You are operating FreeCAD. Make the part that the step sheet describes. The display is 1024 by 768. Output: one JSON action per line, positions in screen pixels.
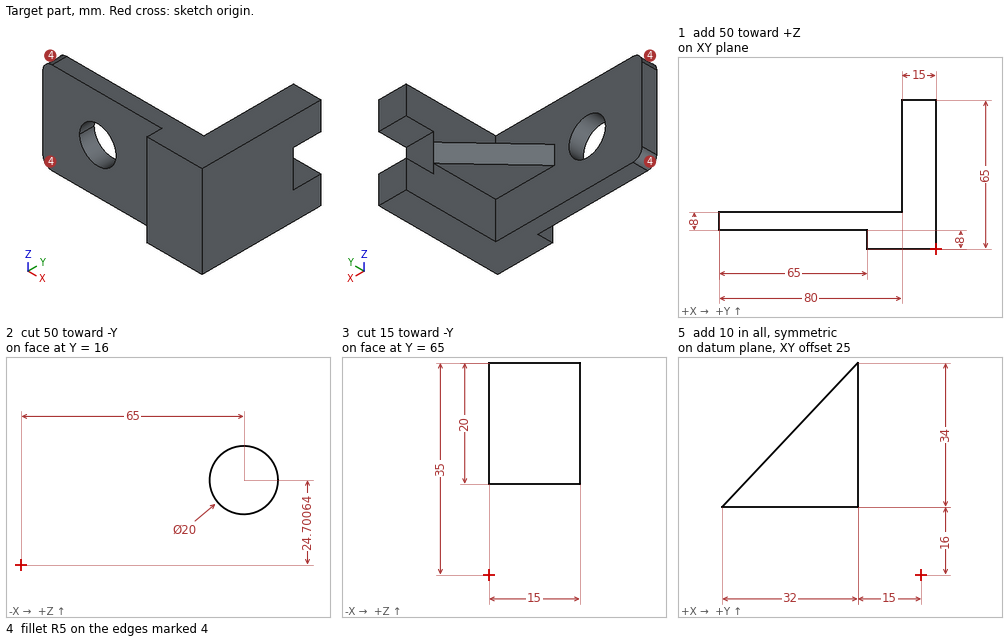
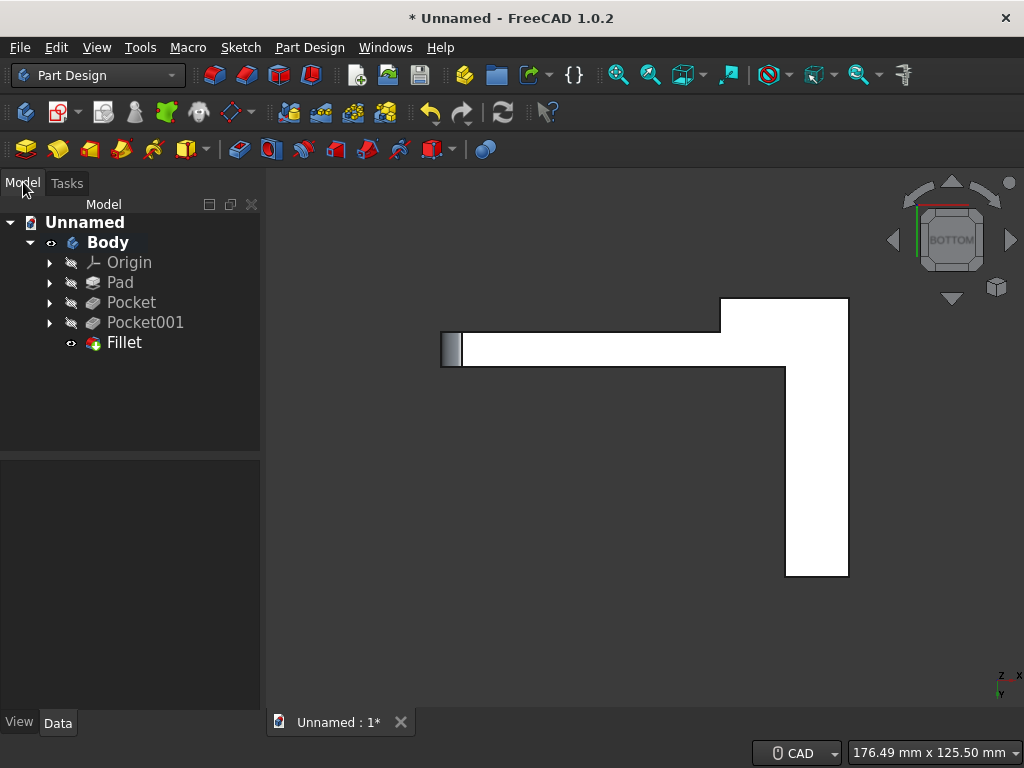
{"action": "left_click", "coordinate": [50, 263]}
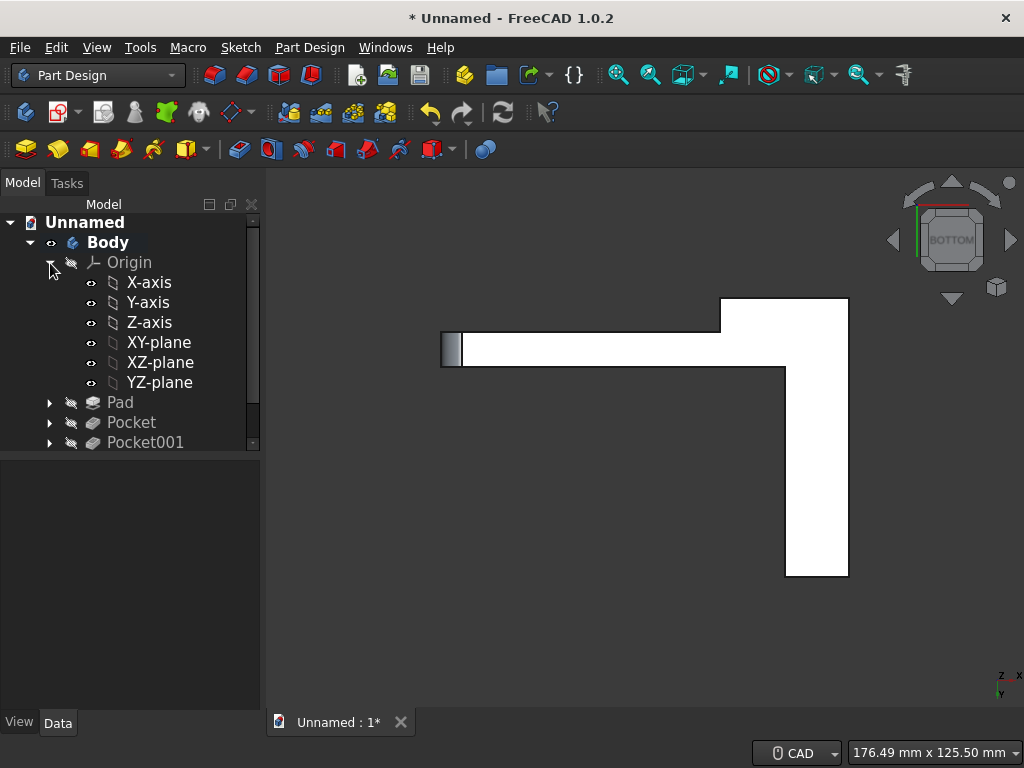
{"action": "left_click", "coordinate": [136, 343]}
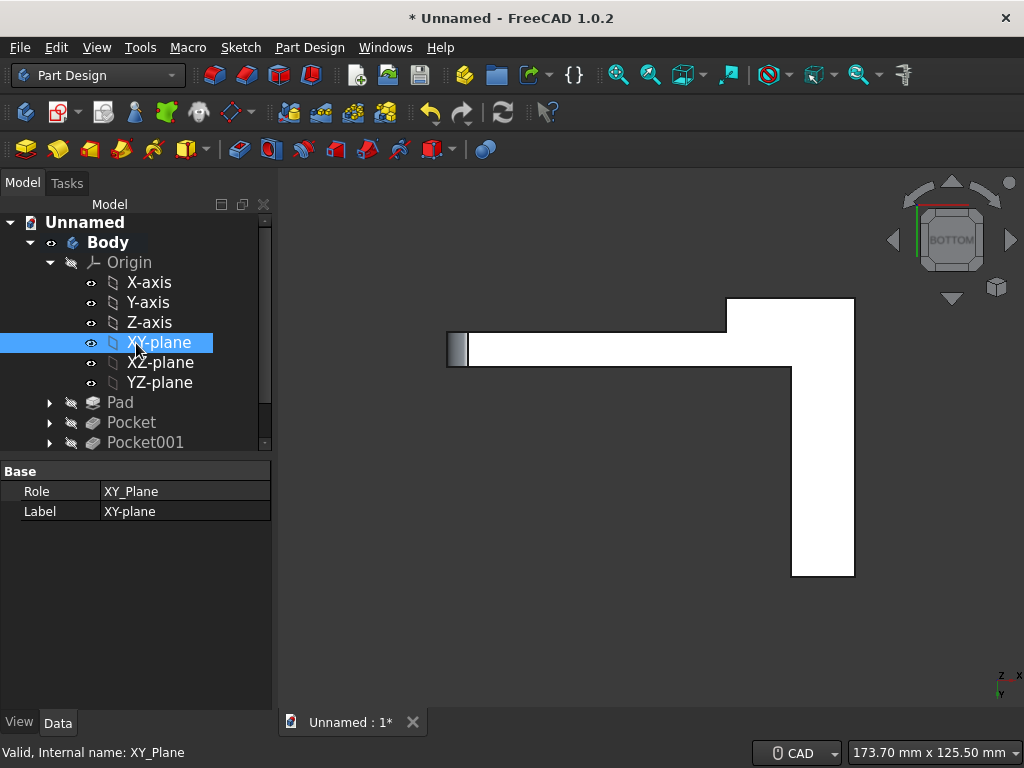
{"action": "left_click", "coordinate": [232, 112]}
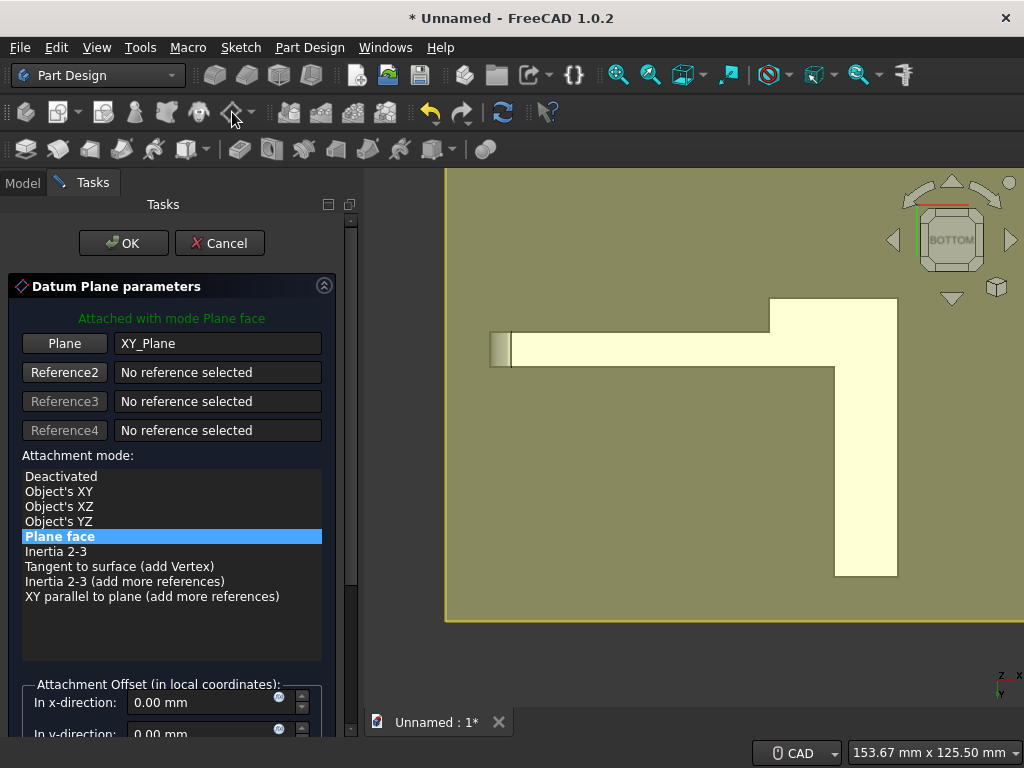
{"action": "scroll", "coordinate": [351, 475], "scroll_direction": "down", "scroll_amount": 2}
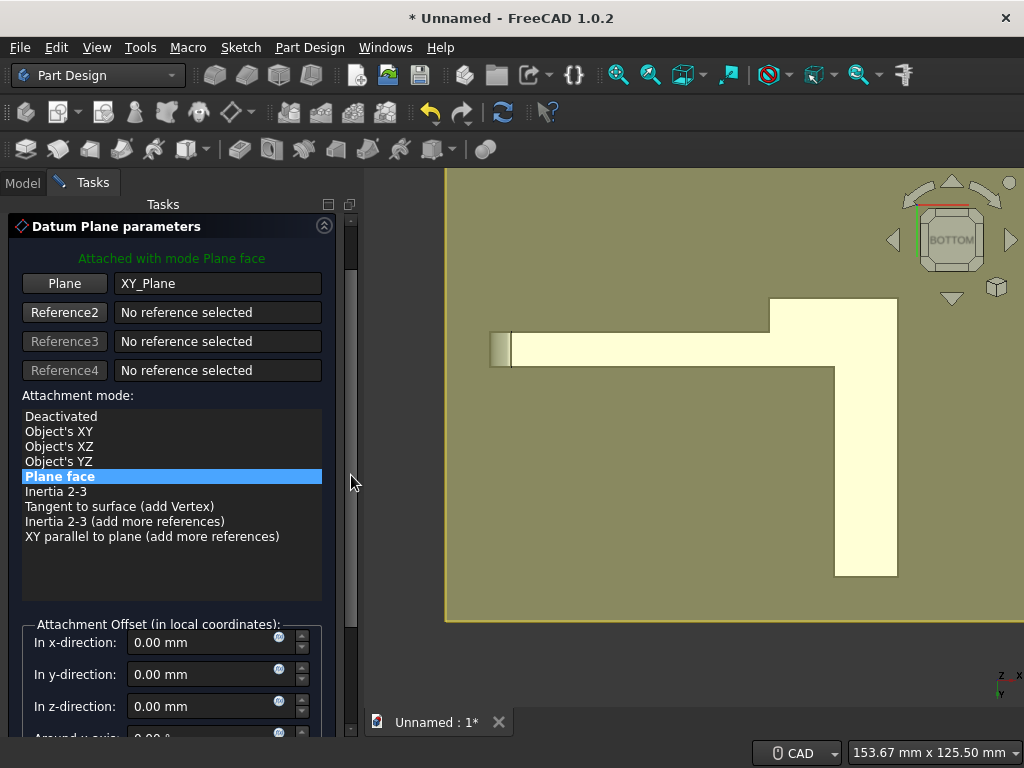
{"action": "triple_click", "coordinate": [210, 646]}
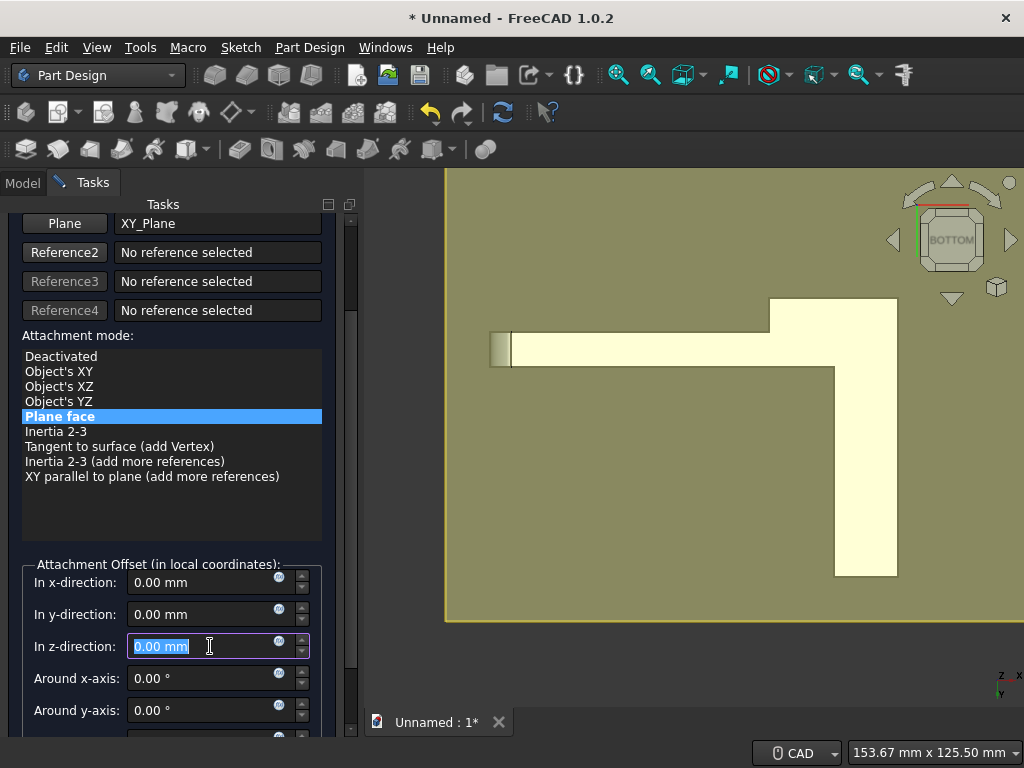
{"action": "type", "text": "25"}
{"action": "key", "text": "Tab"}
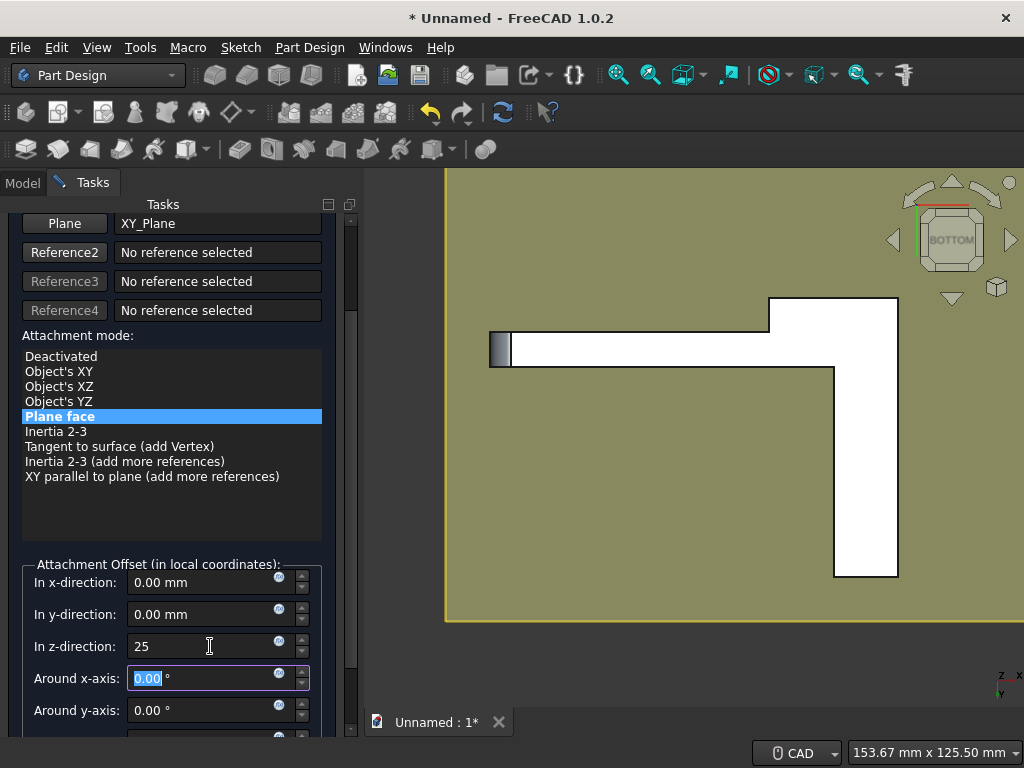
{"action": "scroll", "coordinate": [351, 475], "scroll_direction": "up", "scroll_amount": 3}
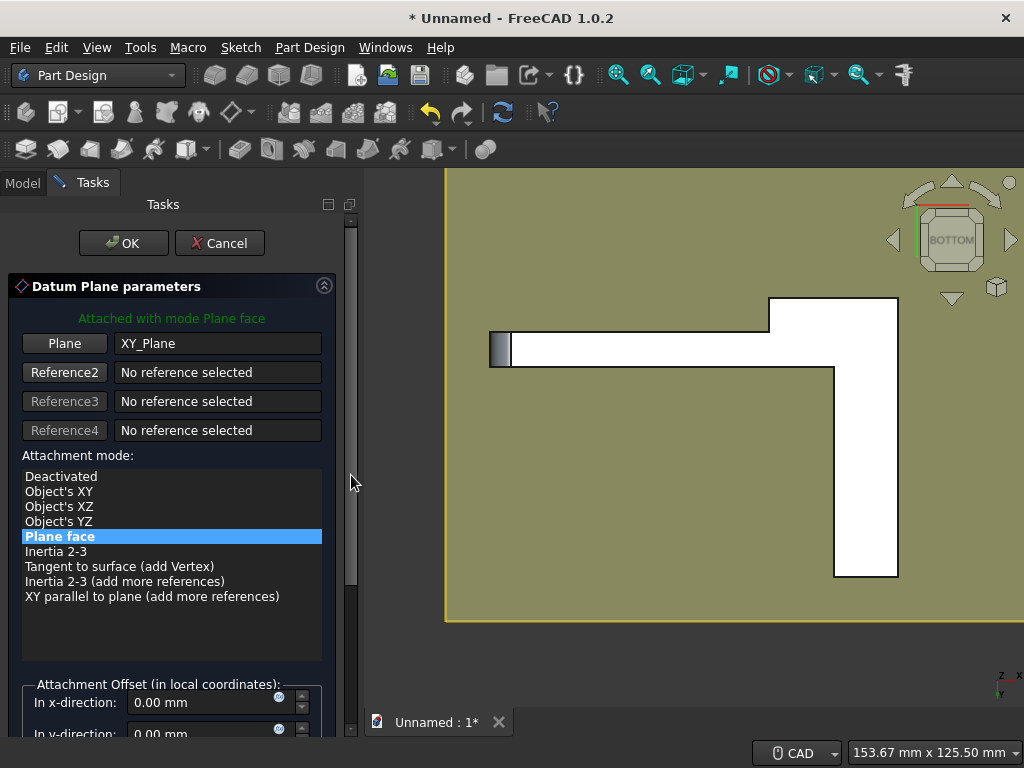
{"action": "left_click", "coordinate": [124, 243]}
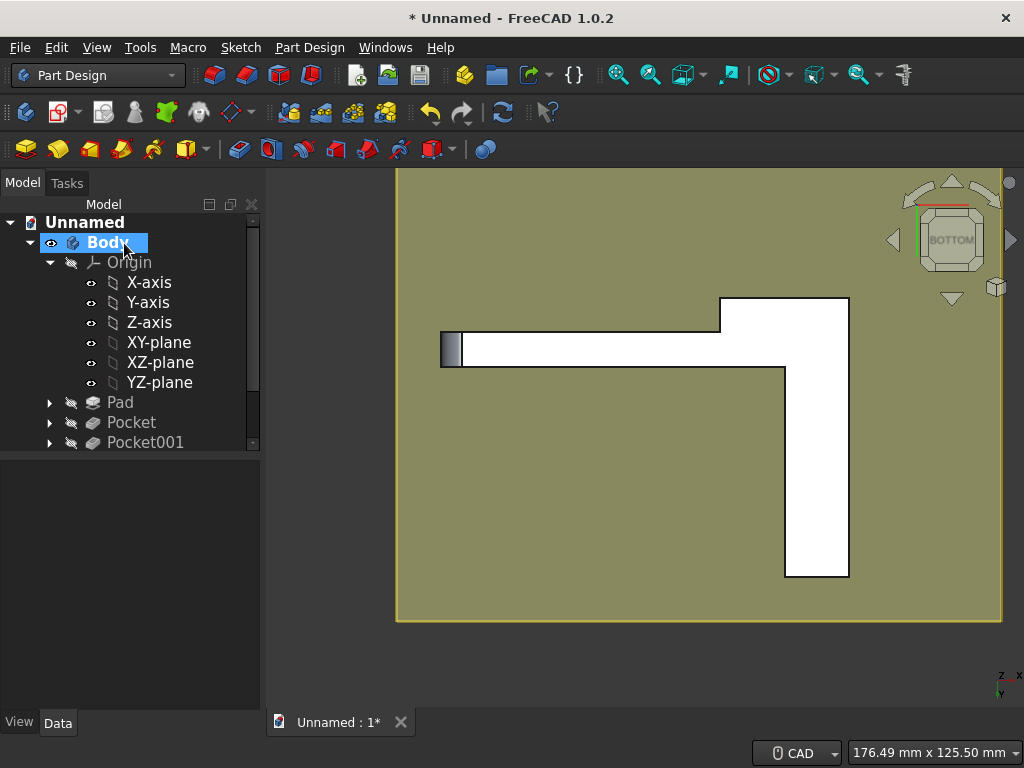
{"action": "scroll", "coordinate": [100, 338], "scroll_direction": "down", "scroll_amount": 3}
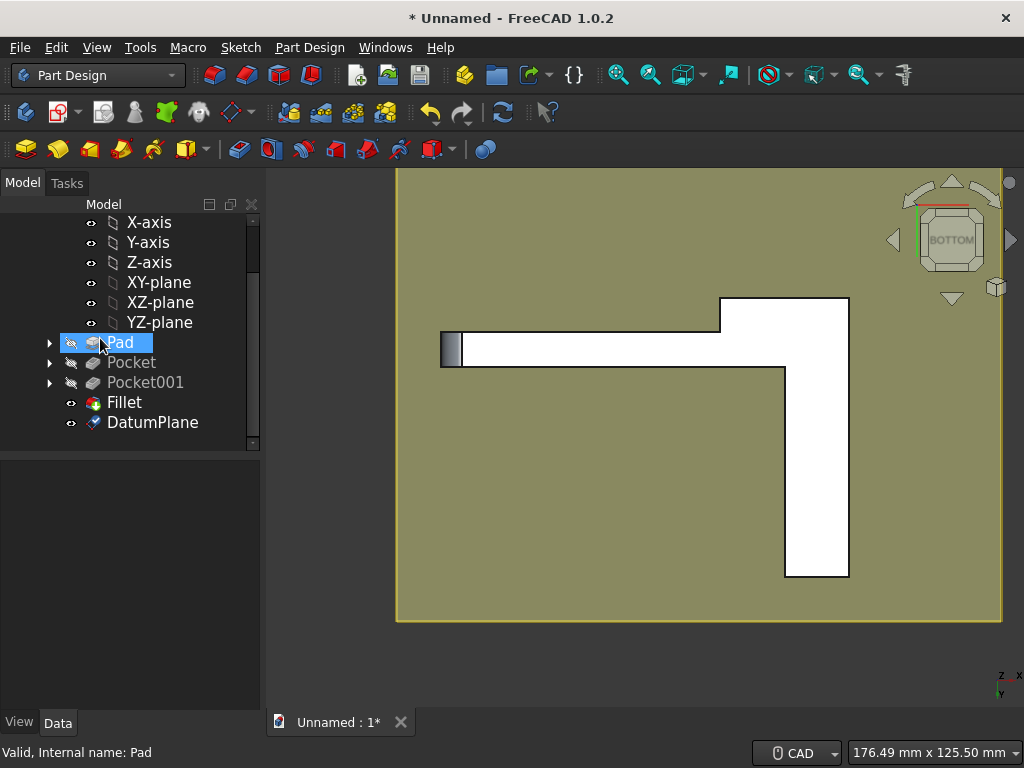
{"action": "left_click", "coordinate": [116, 423]}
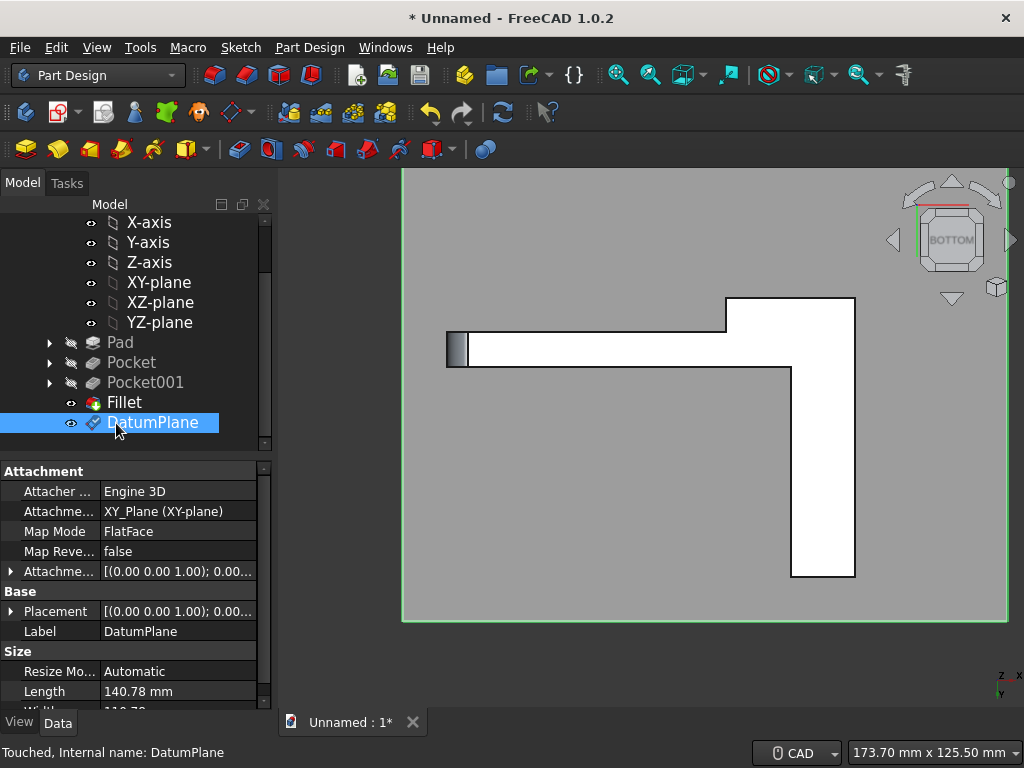
{"action": "left_click", "coordinate": [58, 112]}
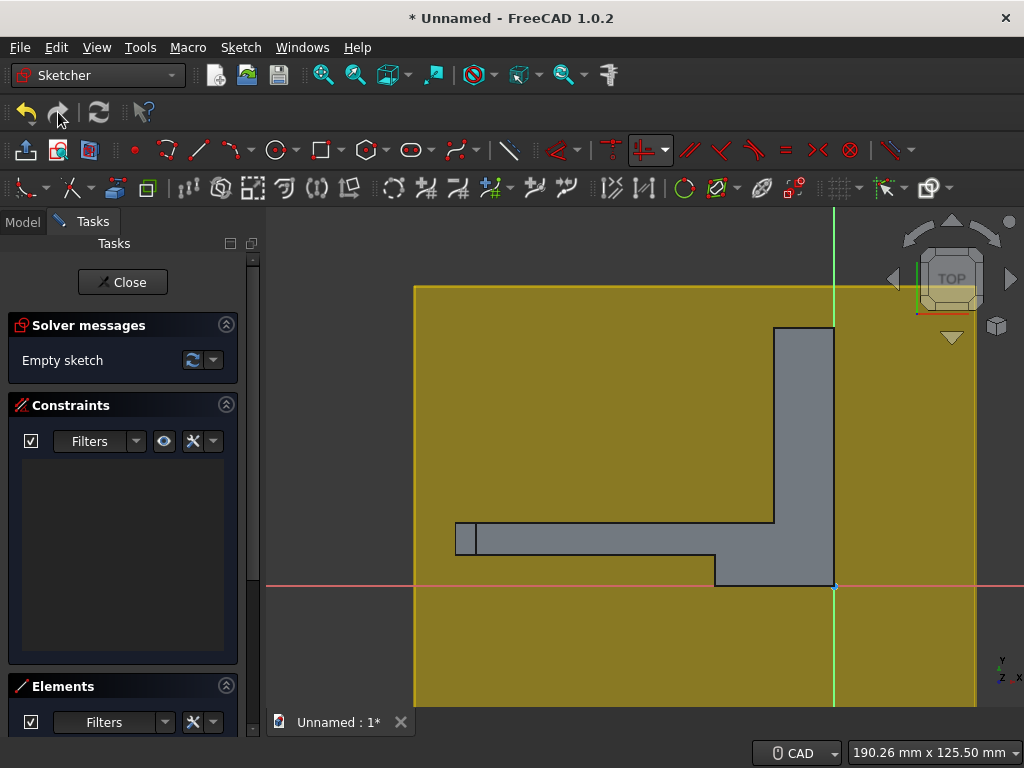
{"action": "left_click", "coordinate": [90, 150]}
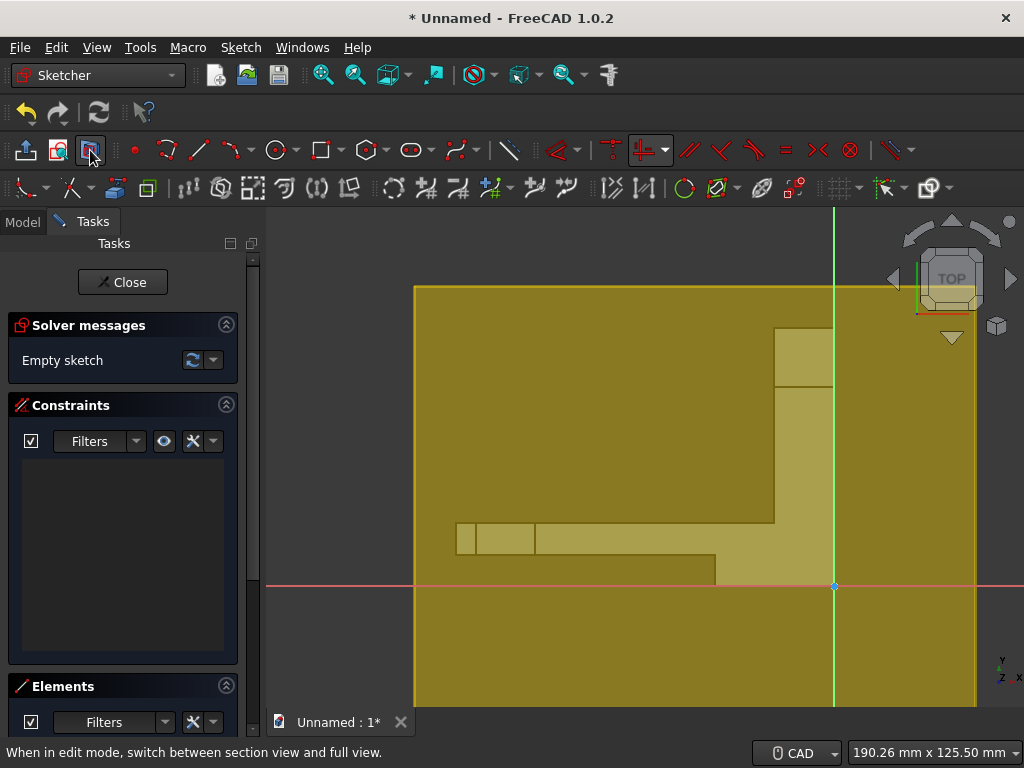
{"action": "scroll", "coordinate": [859, 548], "scroll_direction": "up", "scroll_amount": 2}